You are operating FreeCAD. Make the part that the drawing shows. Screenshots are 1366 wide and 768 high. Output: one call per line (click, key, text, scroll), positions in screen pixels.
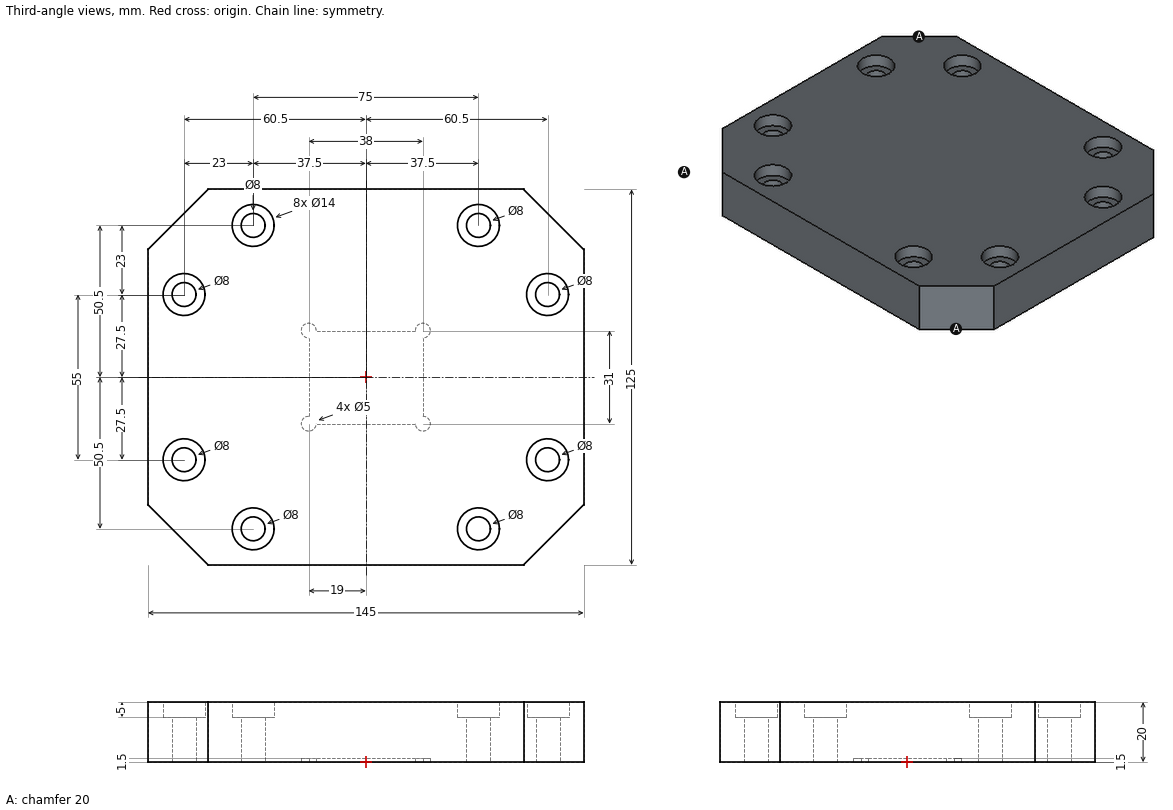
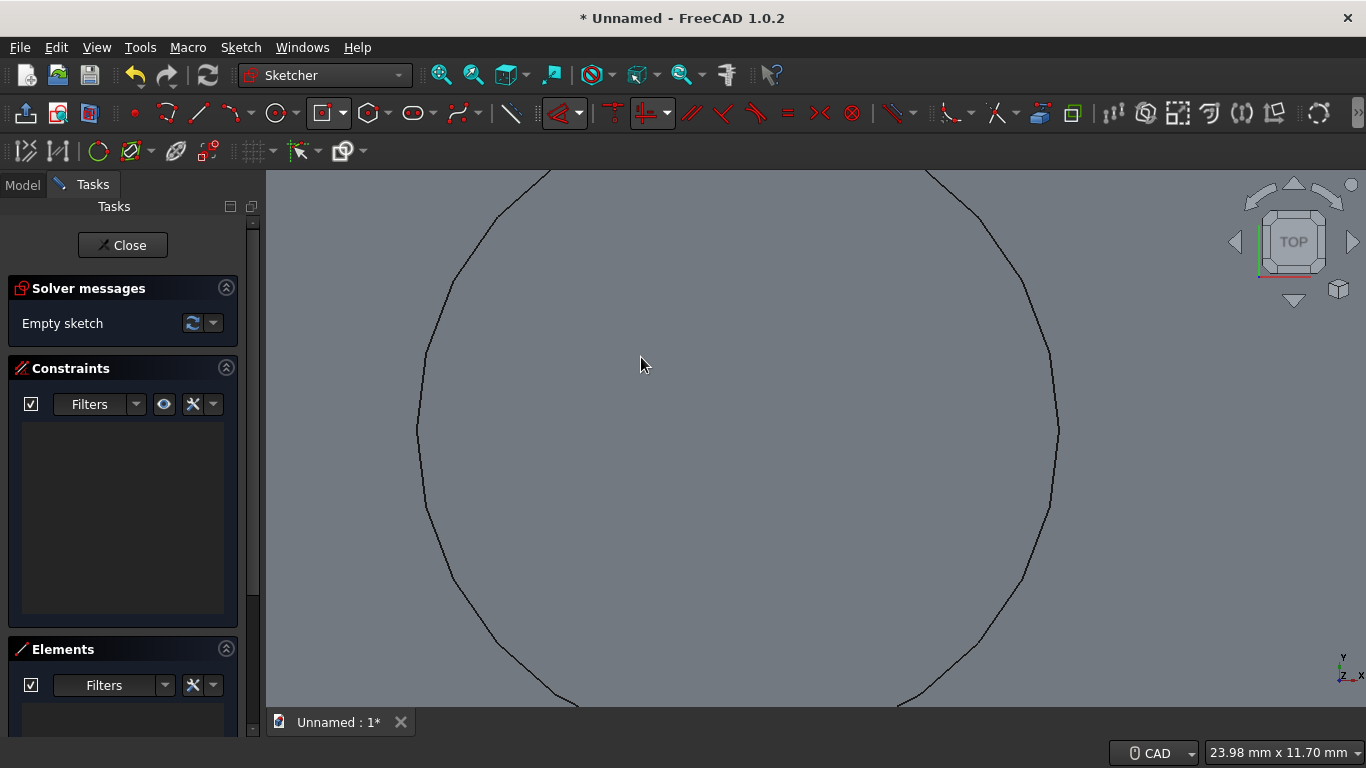
key(g)
key(c)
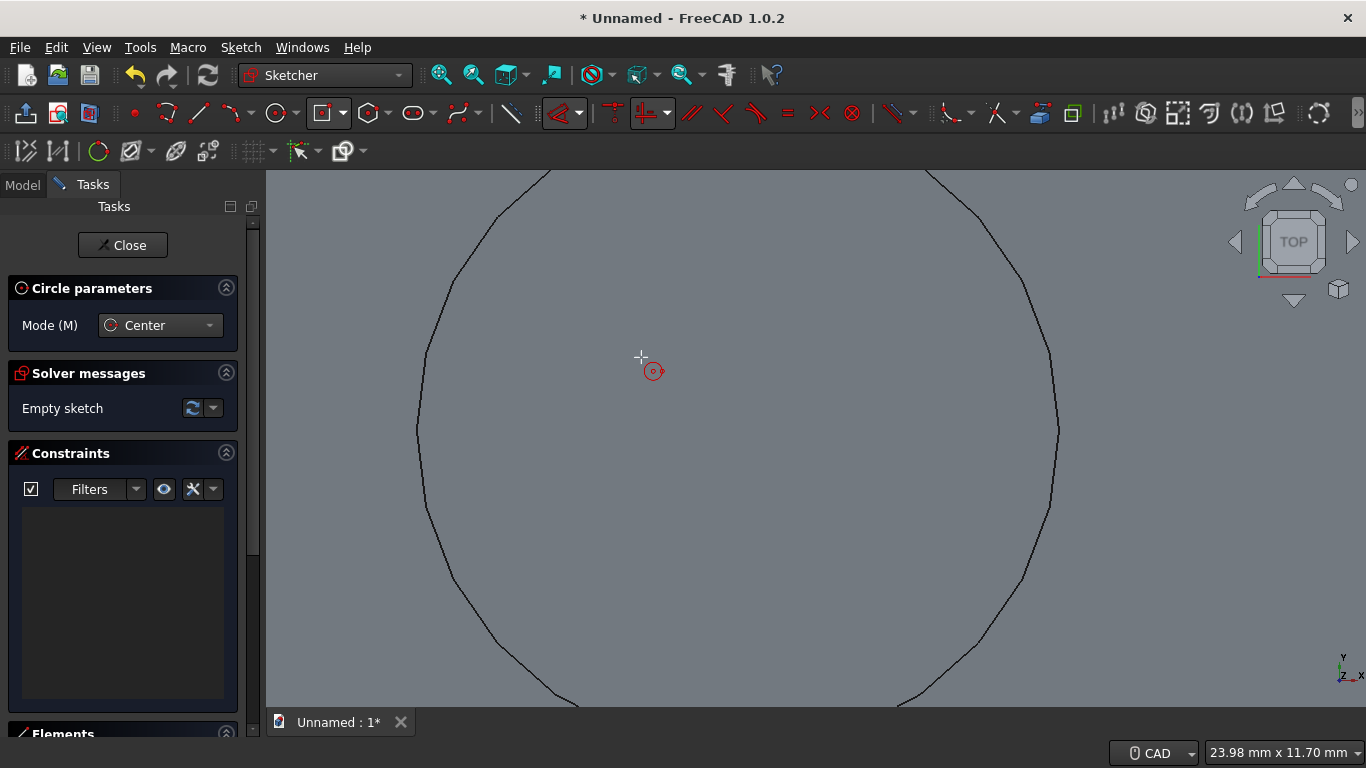
click(738, 430)
click(868, 300)
key(Escape)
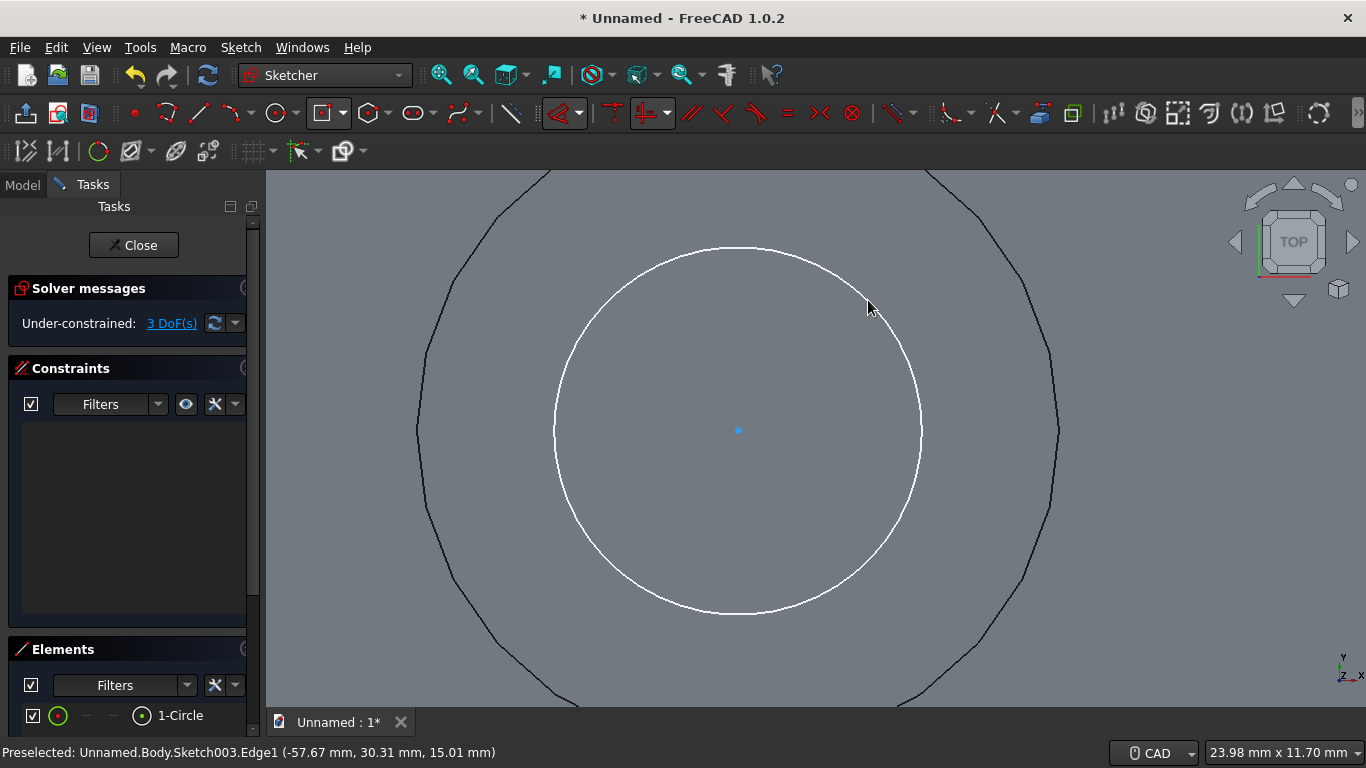
click(868, 301)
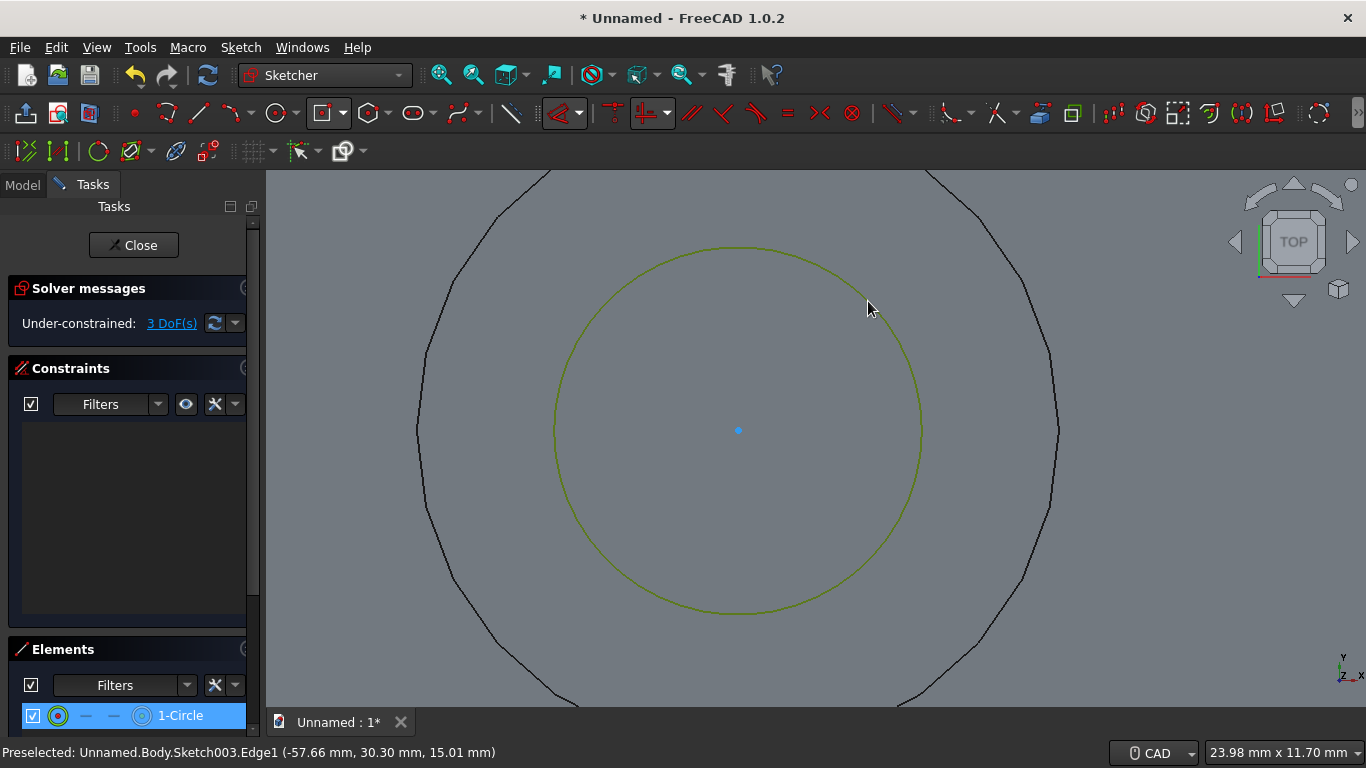
key(k)
key(o)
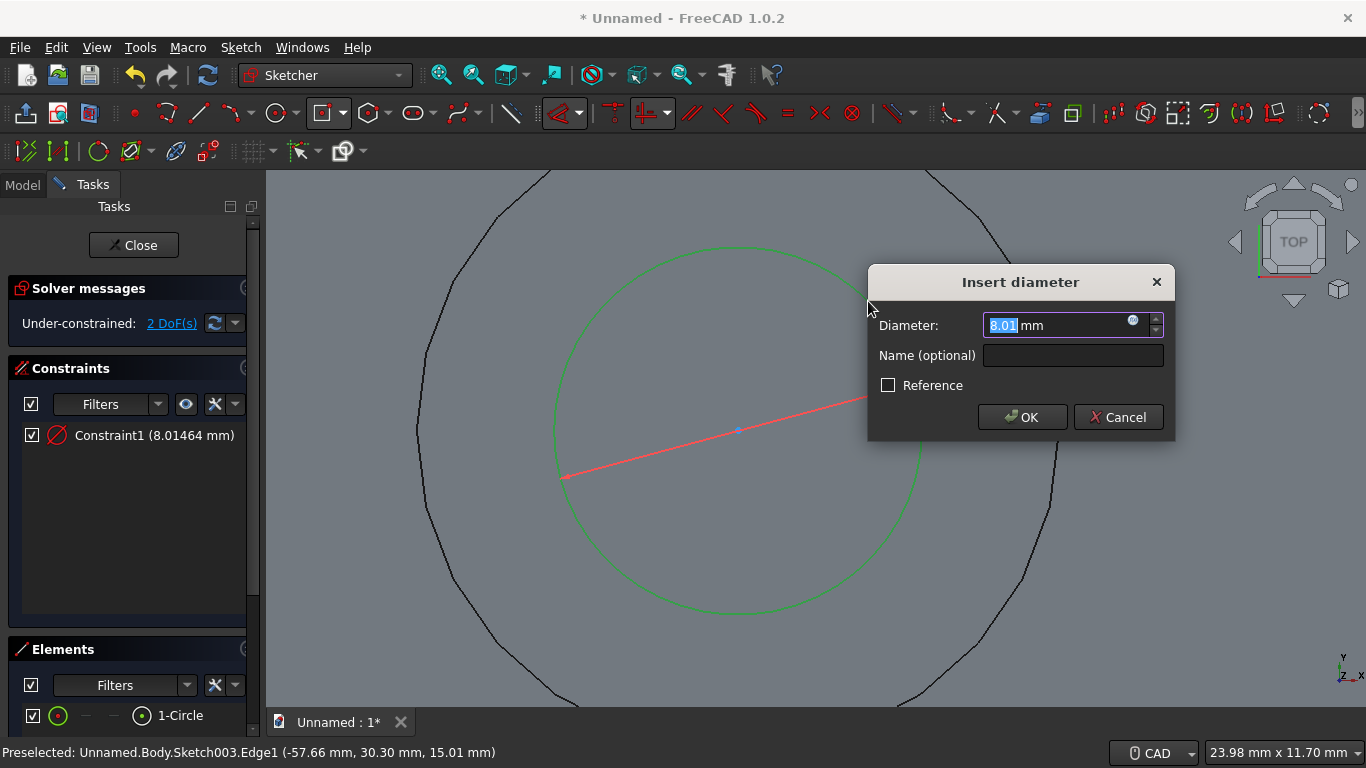
text(8)
key(Return)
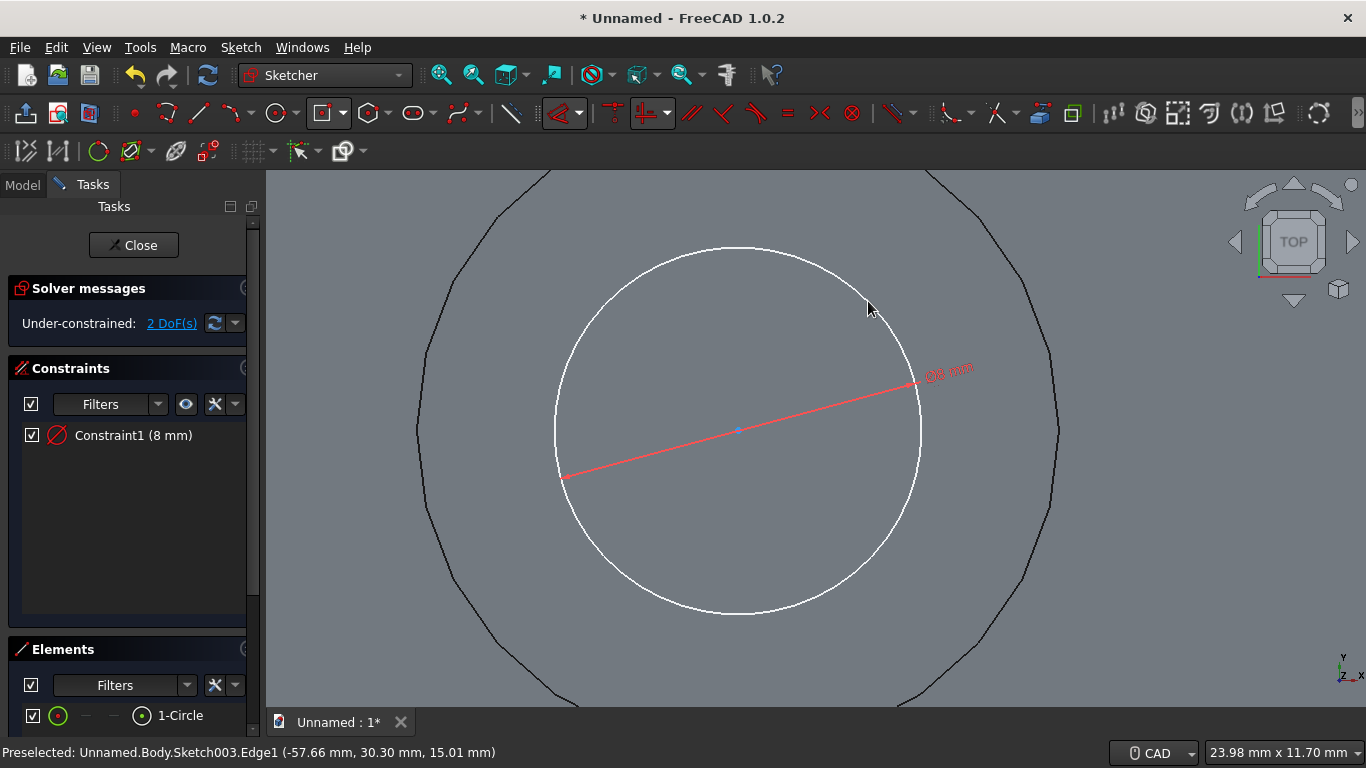
click(738, 431)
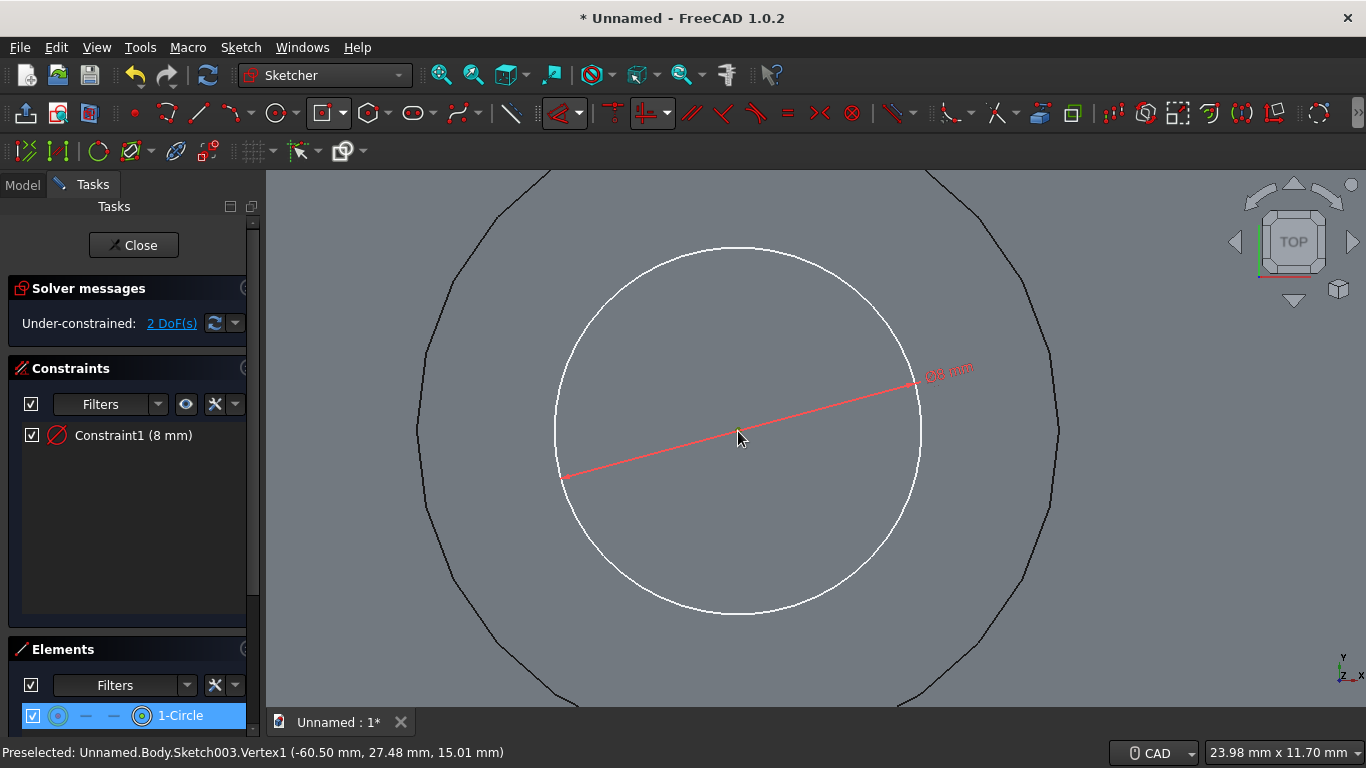
key(l)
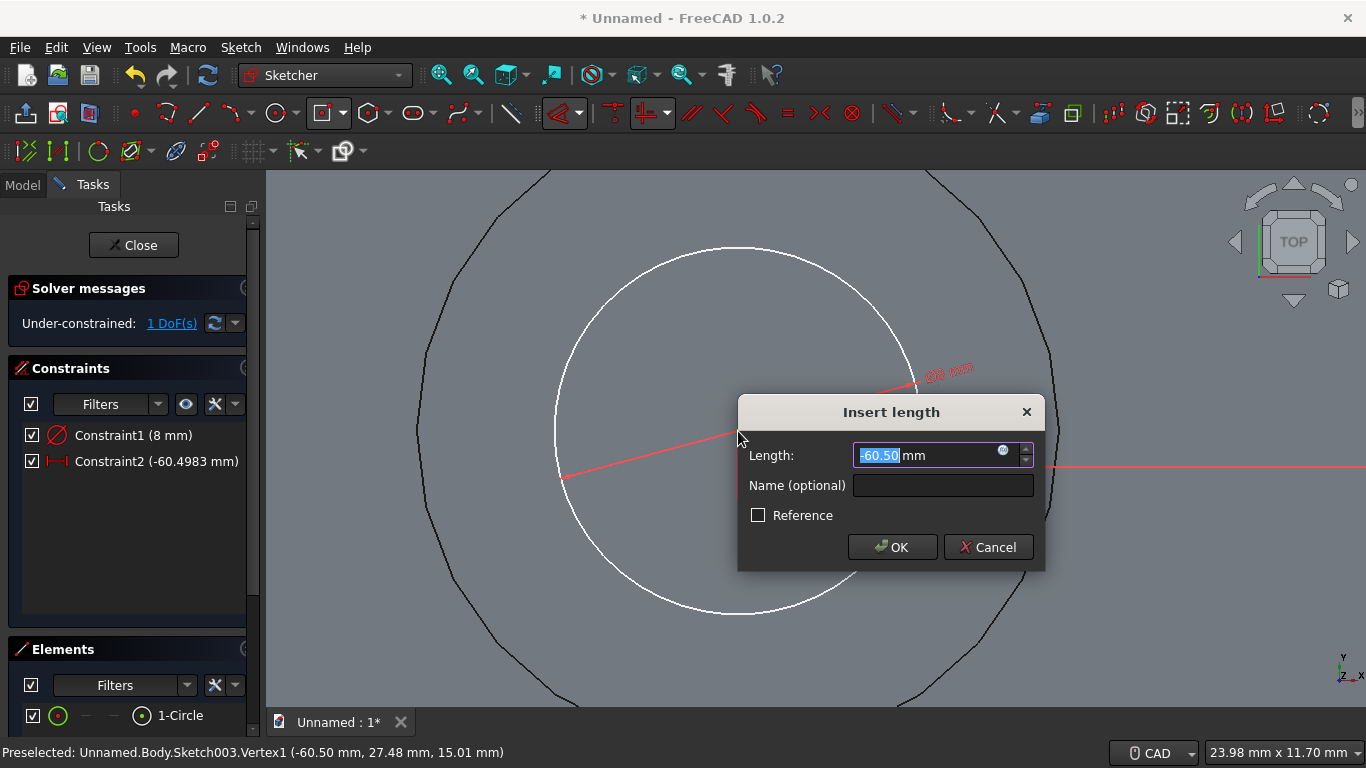
text(-60.5)
key(Return)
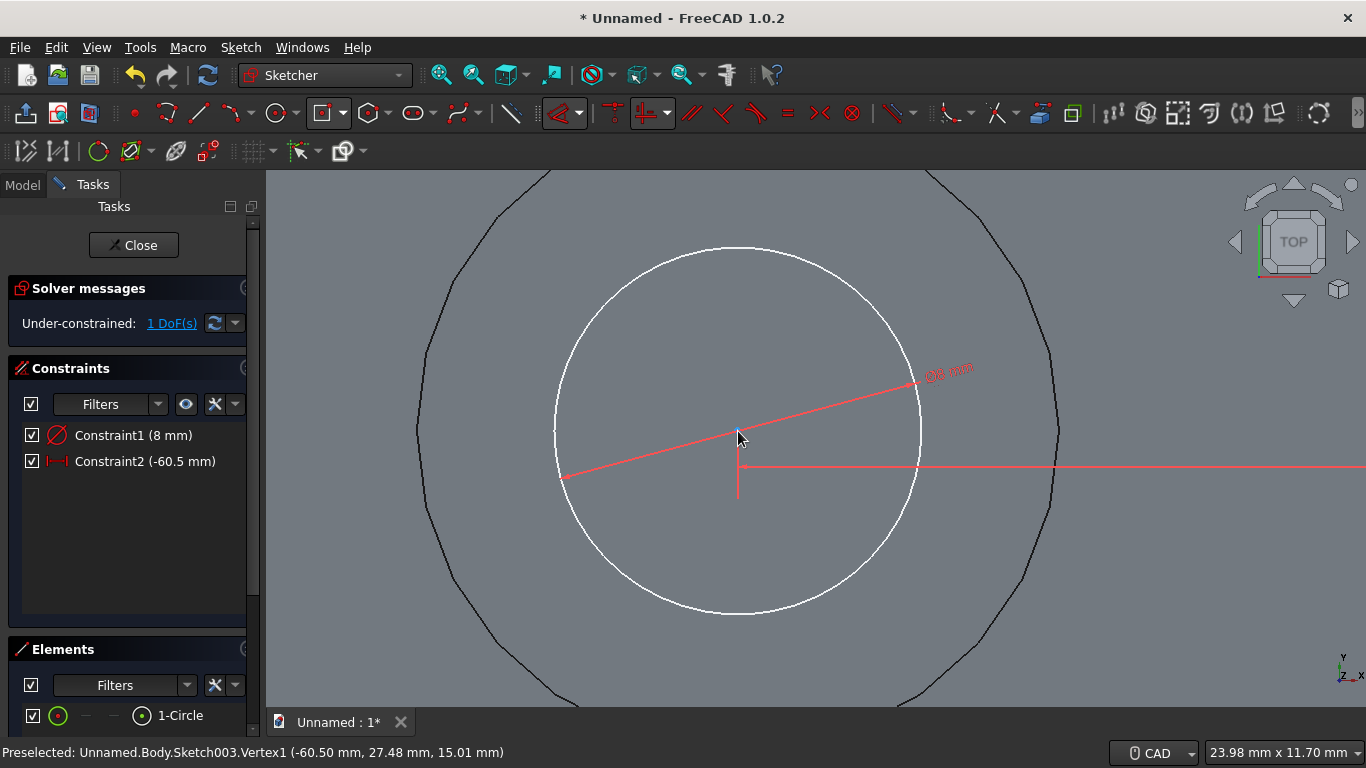
click(738, 431)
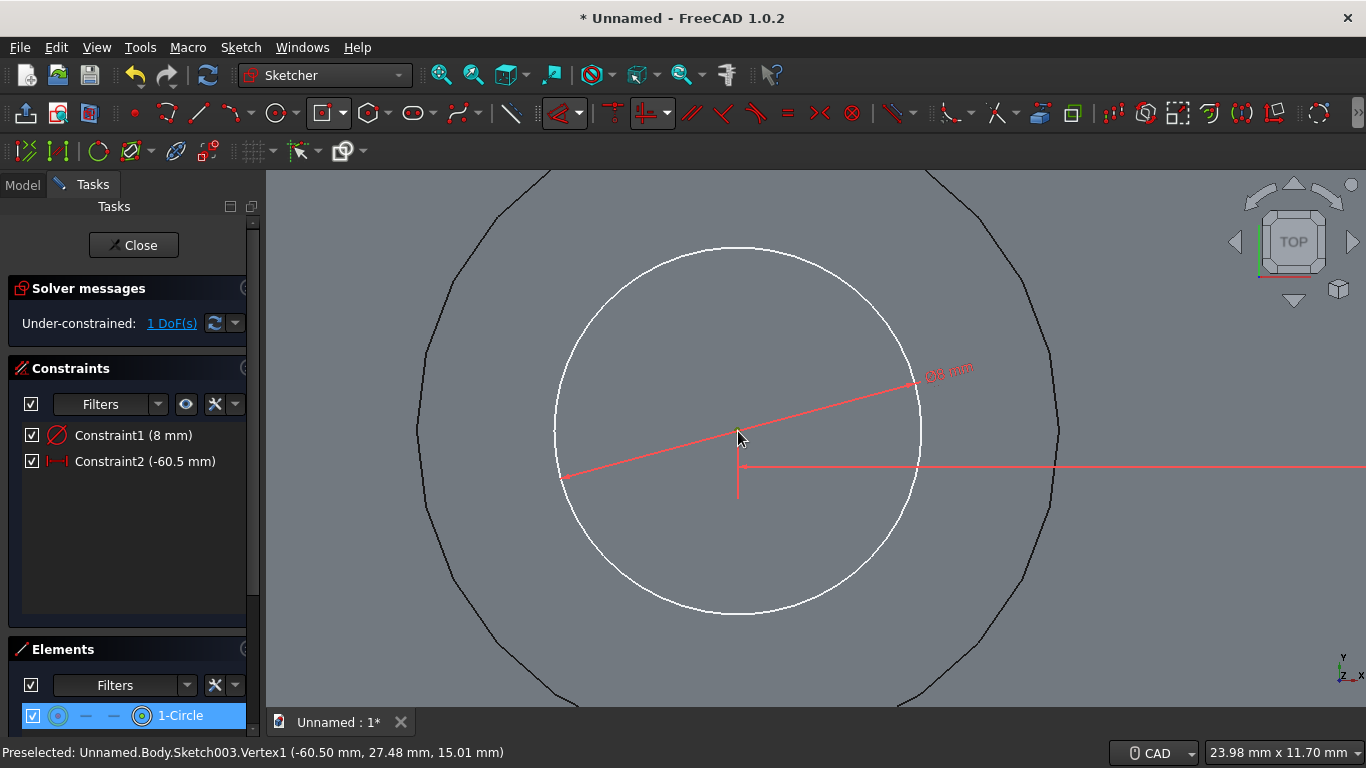
key(i)